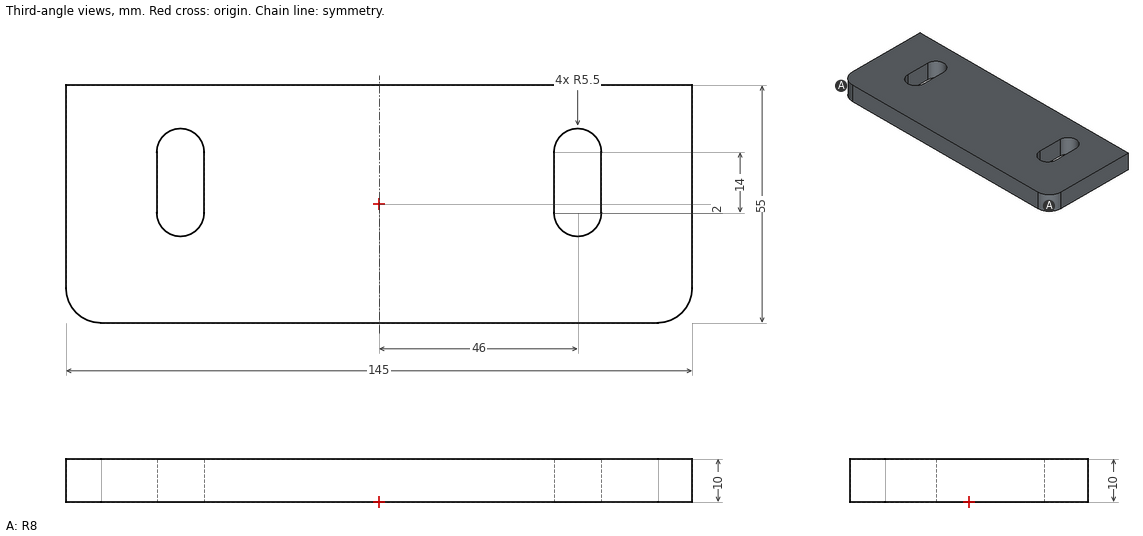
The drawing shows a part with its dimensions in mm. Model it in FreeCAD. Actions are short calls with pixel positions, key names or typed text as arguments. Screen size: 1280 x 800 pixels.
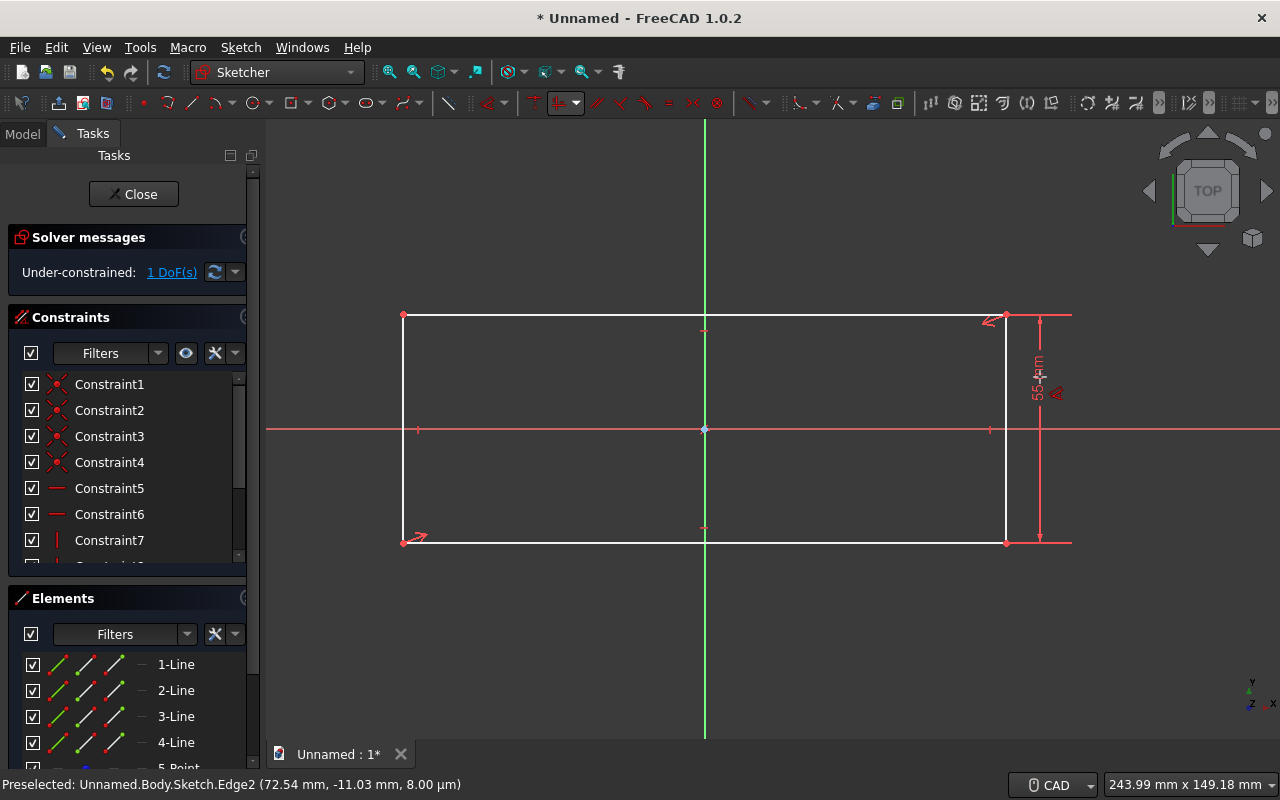
click(584, 543)
click(566, 577)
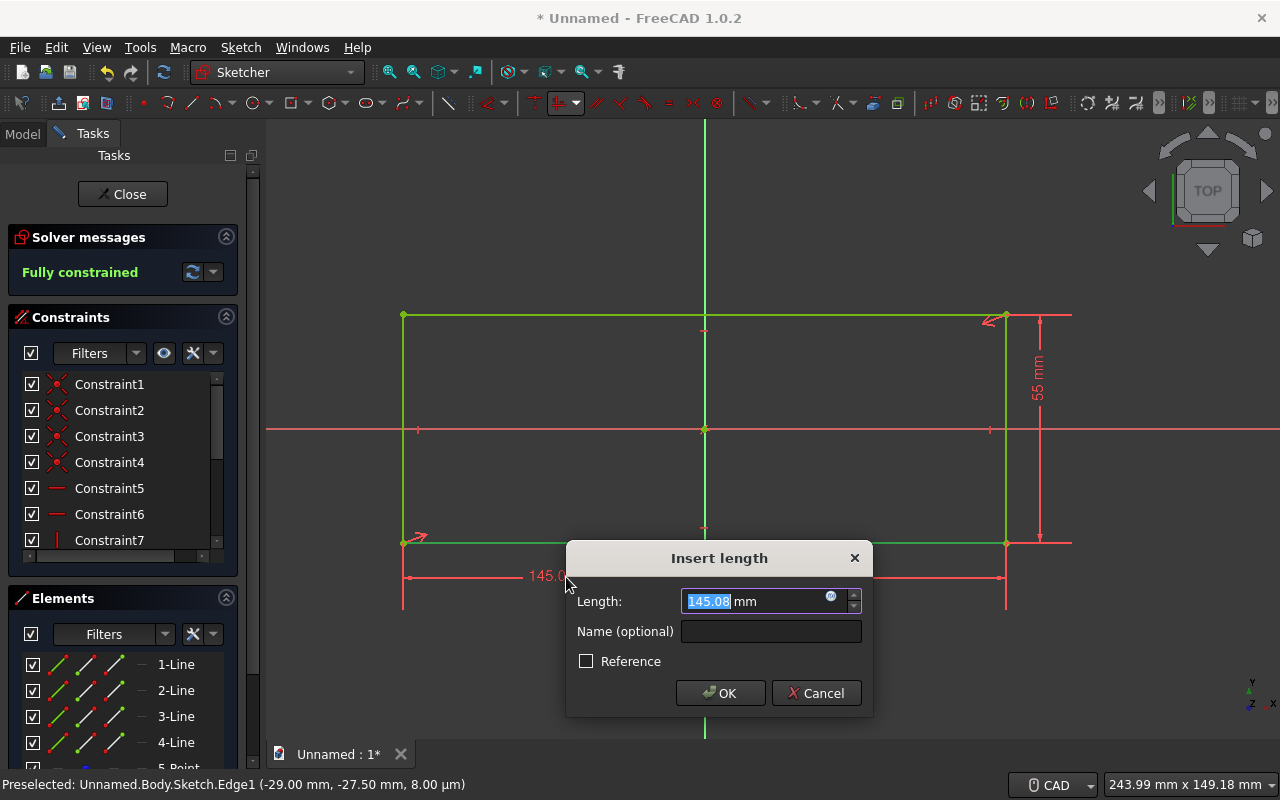
text(145)
key(Return)
key(Escape)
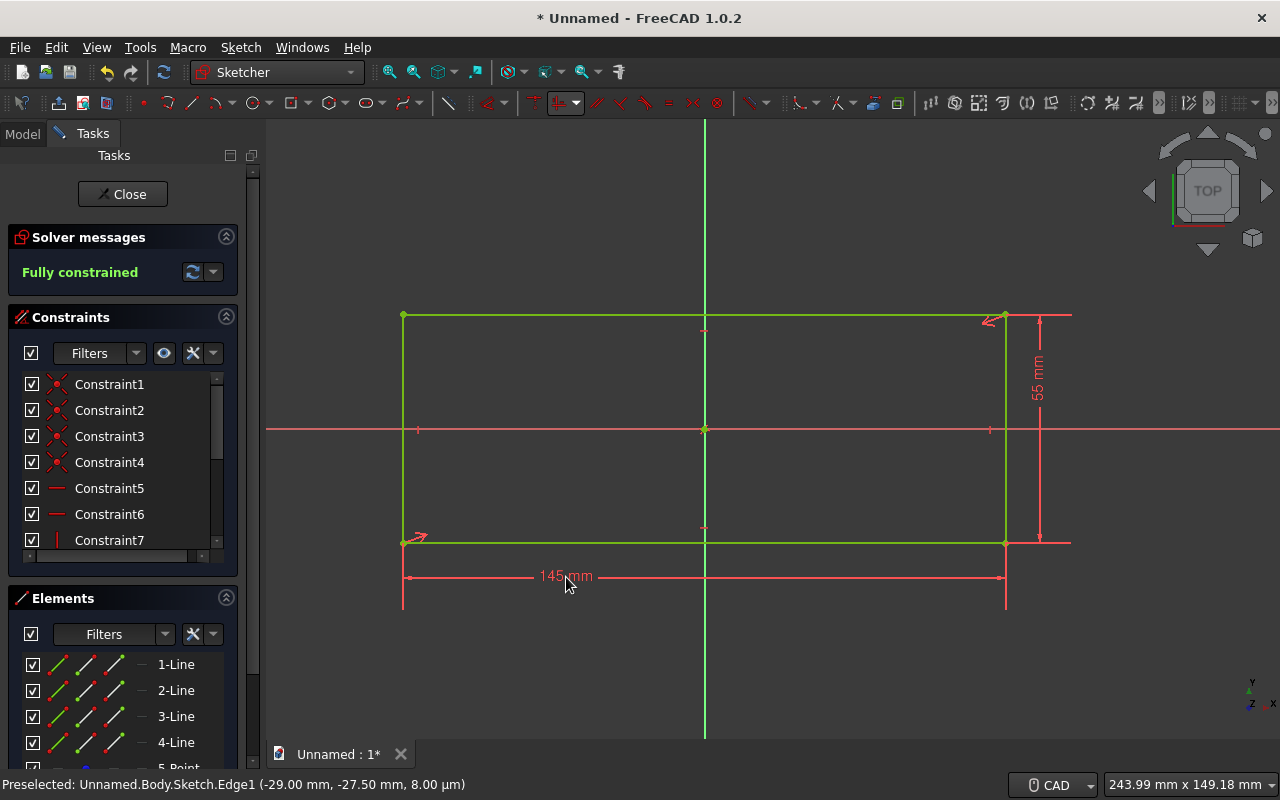
click(123, 194)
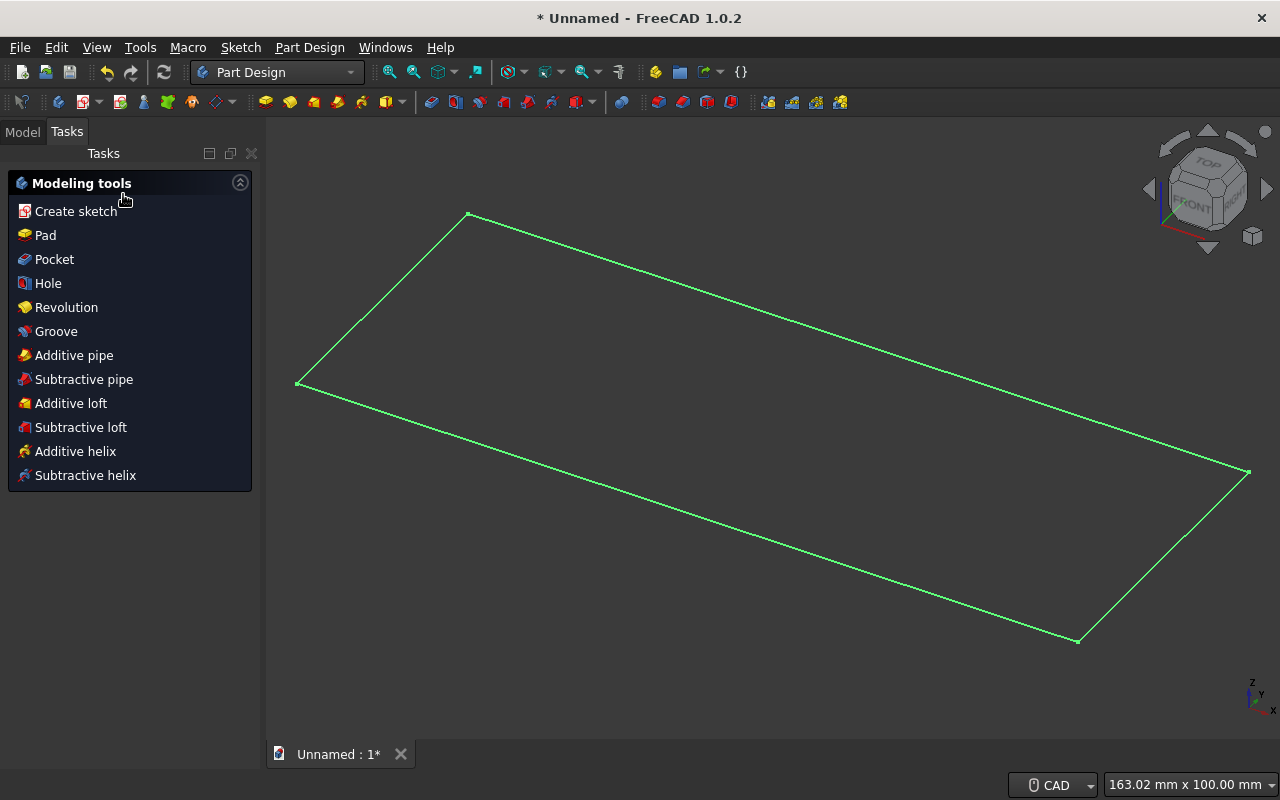
click(266, 102)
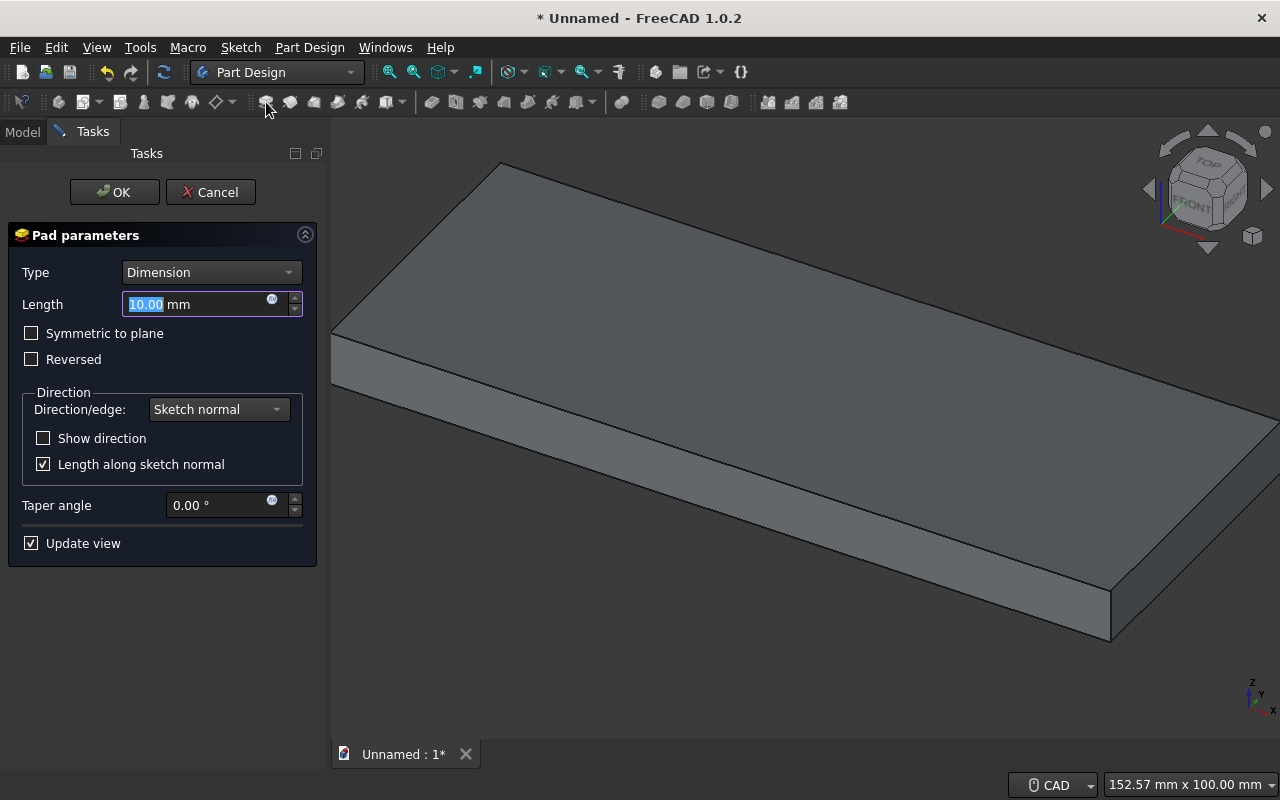
text(10)
key(Tab)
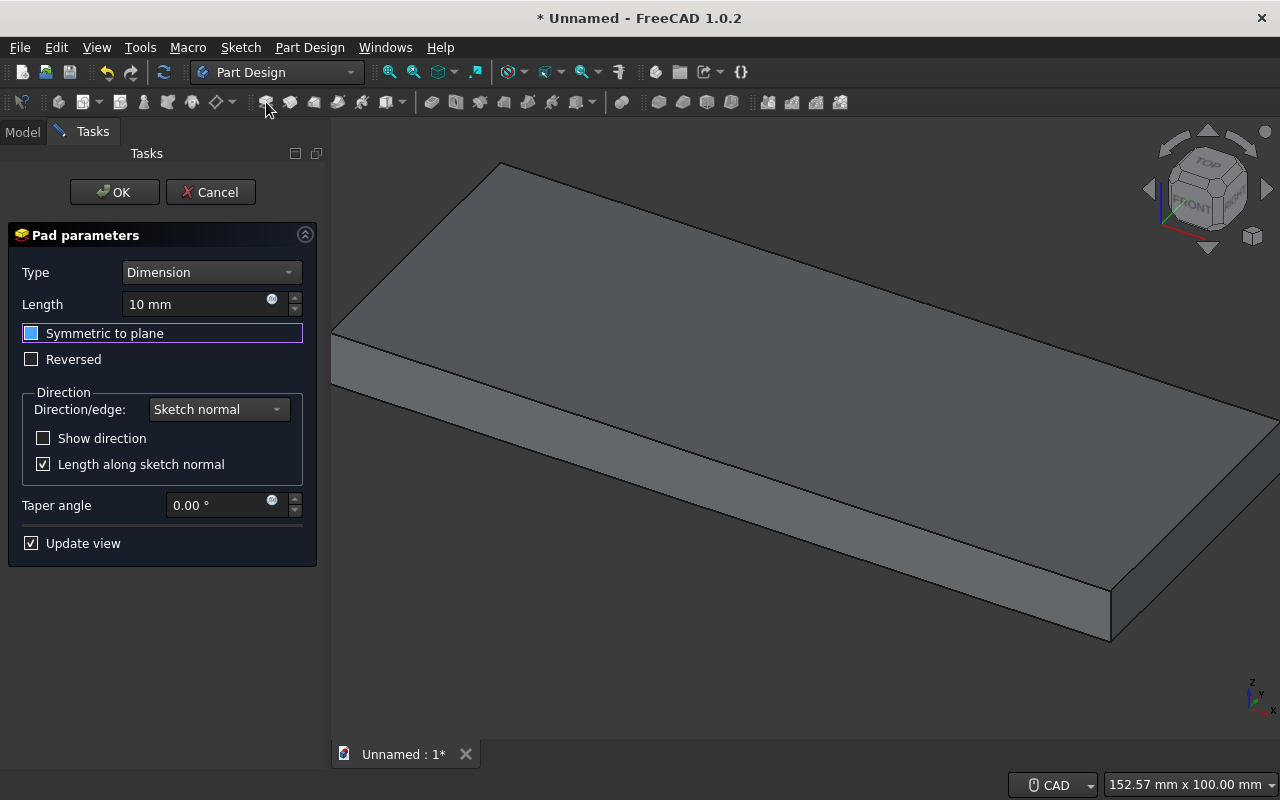
click(115, 192)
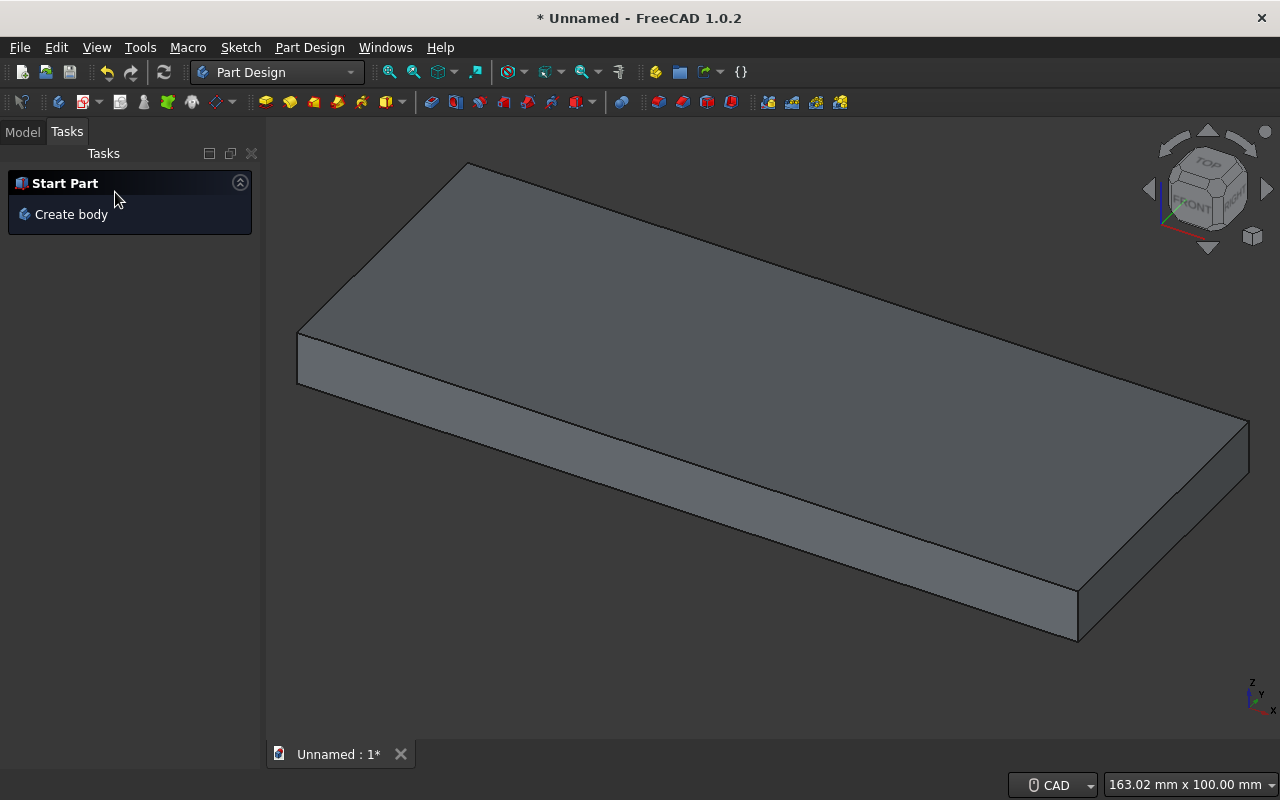
click(1078, 616)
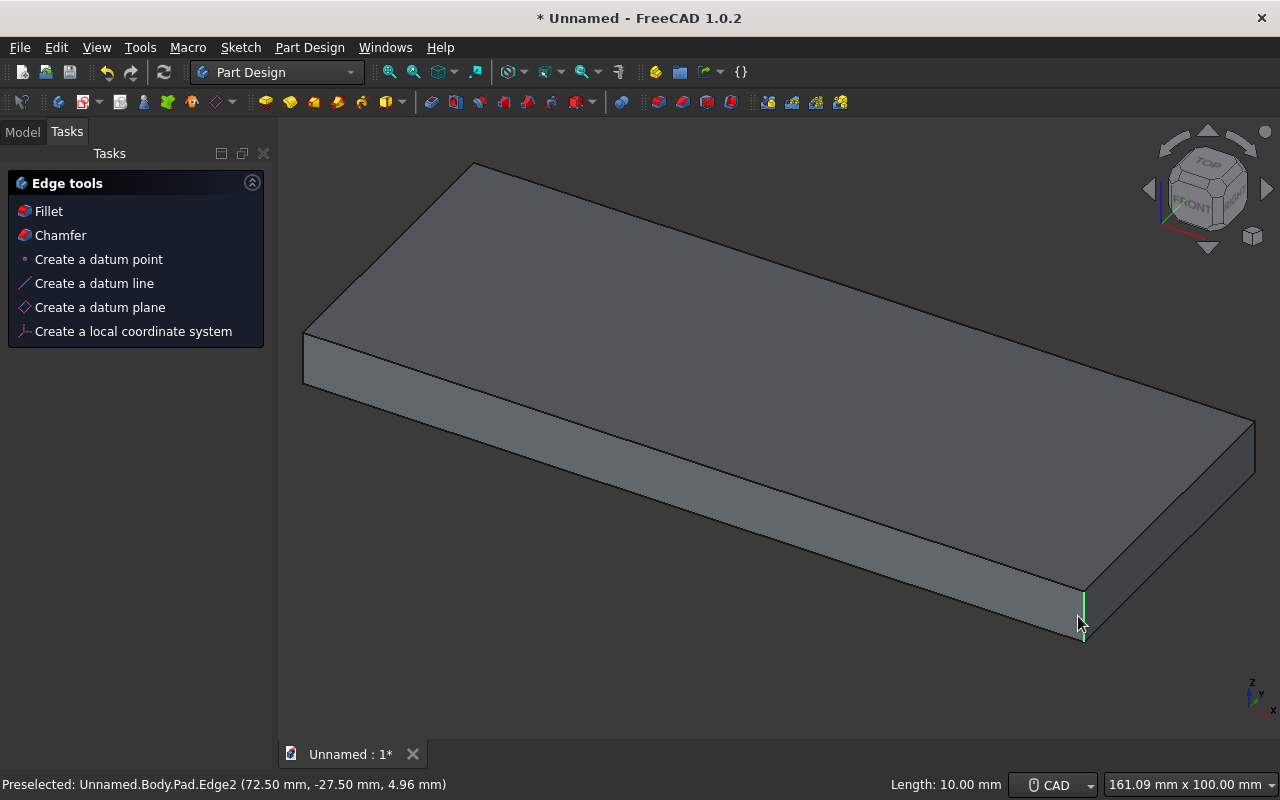
key(0)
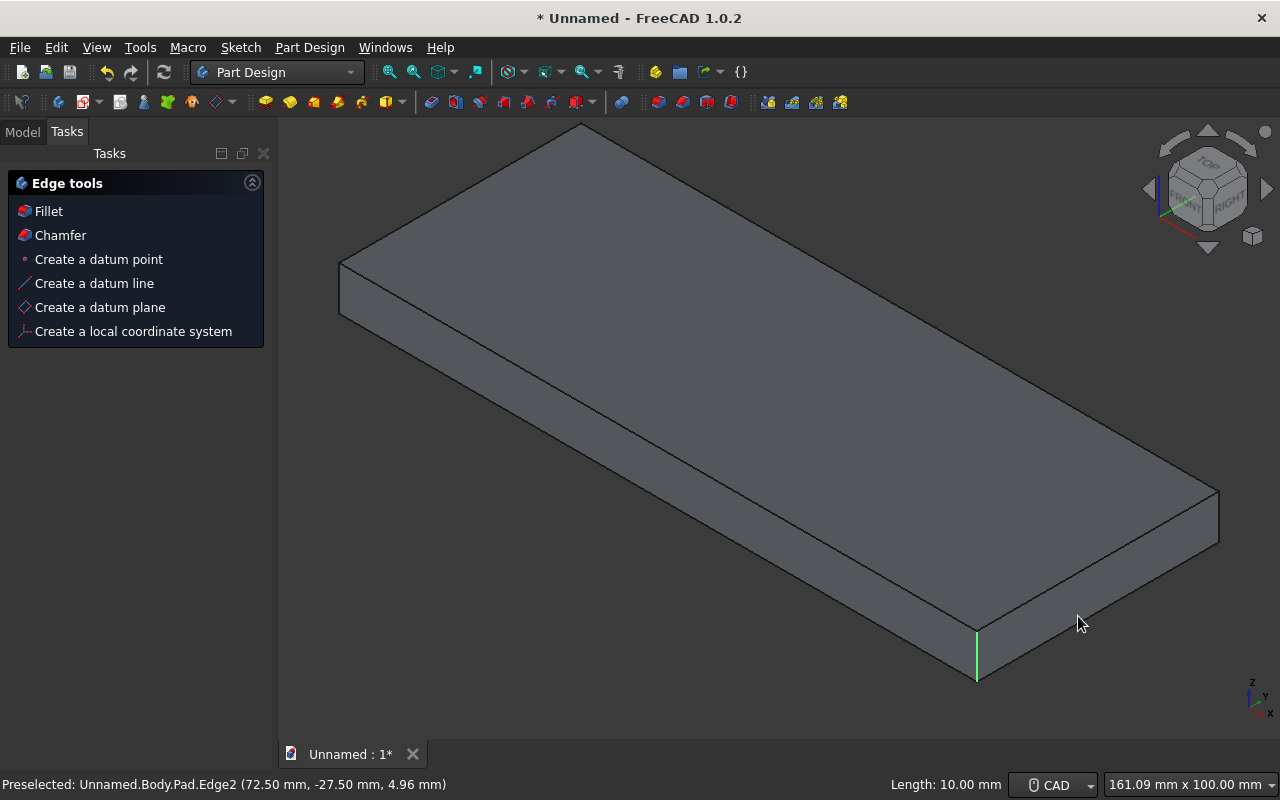
key(2)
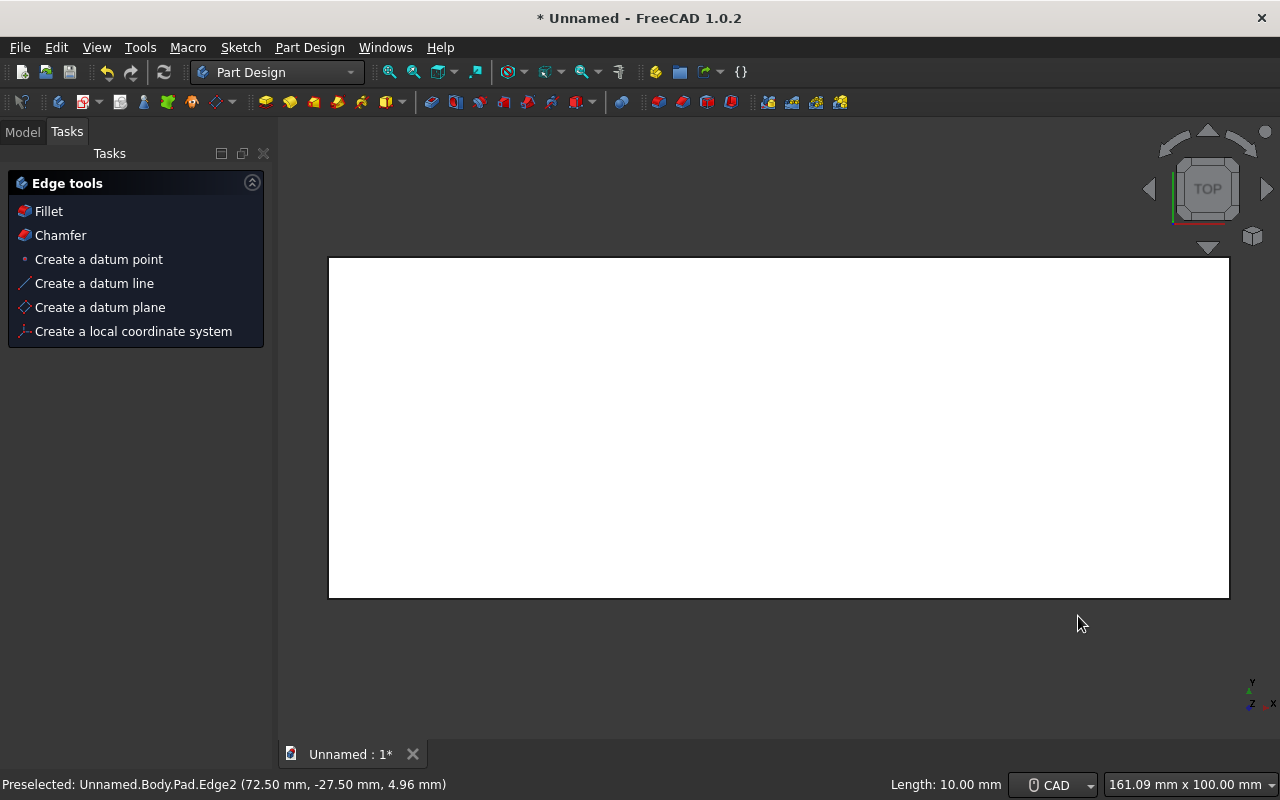
key(1)